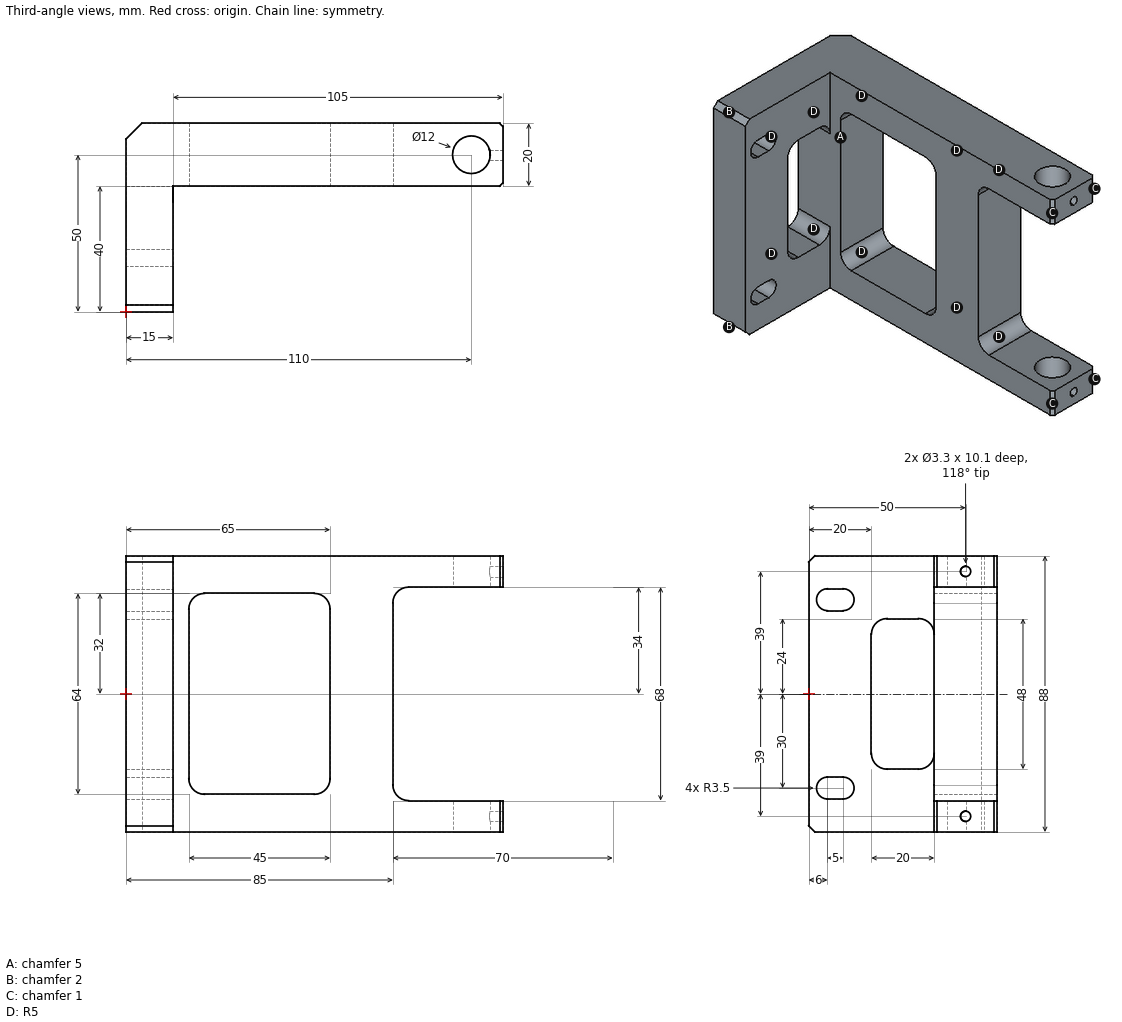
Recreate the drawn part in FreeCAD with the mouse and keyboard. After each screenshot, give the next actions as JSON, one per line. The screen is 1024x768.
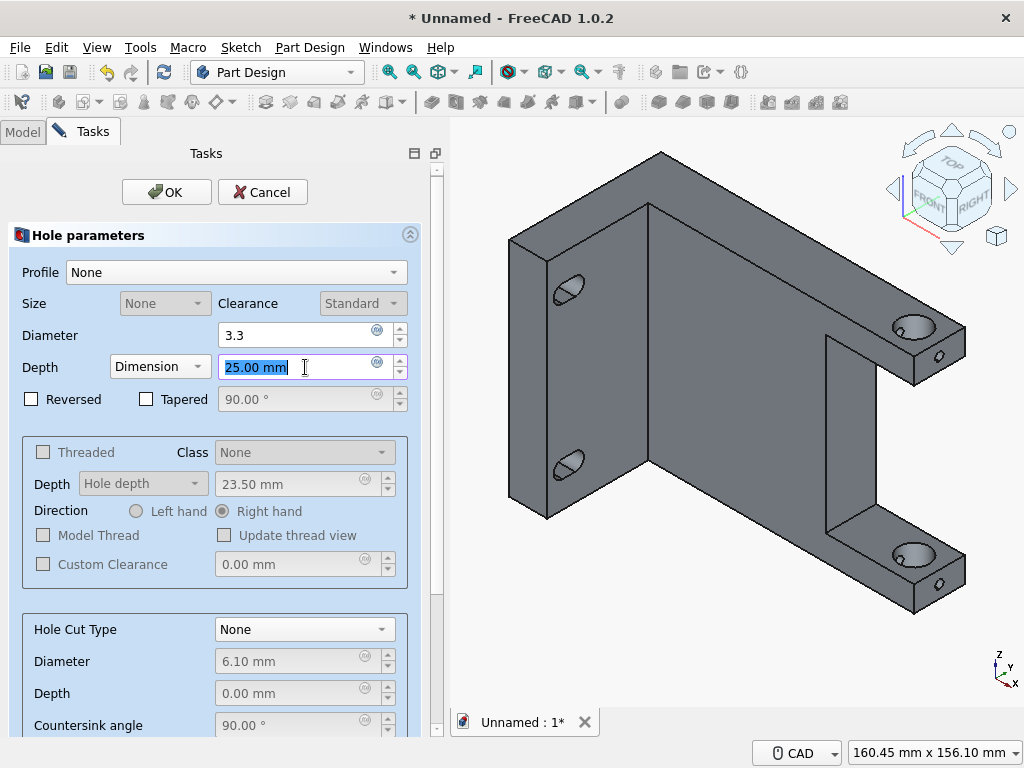
{"action": "type", "text": "10.1"}
{"action": "key", "text": "Tab"}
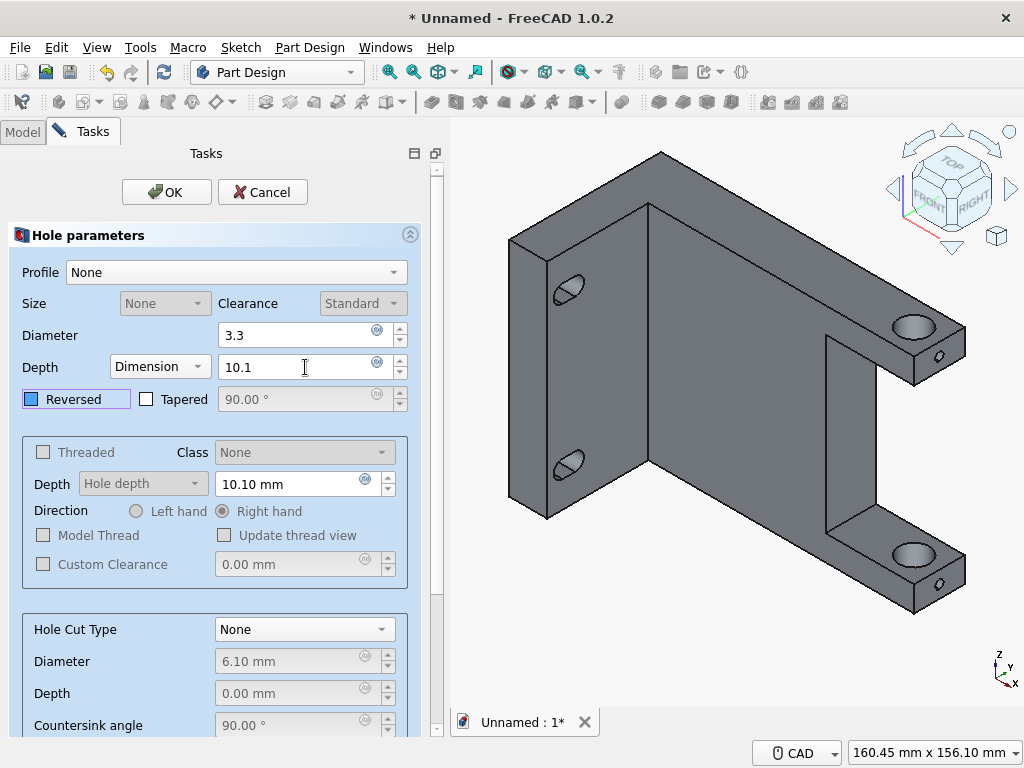
{"action": "left_click", "coordinate": [167, 192]}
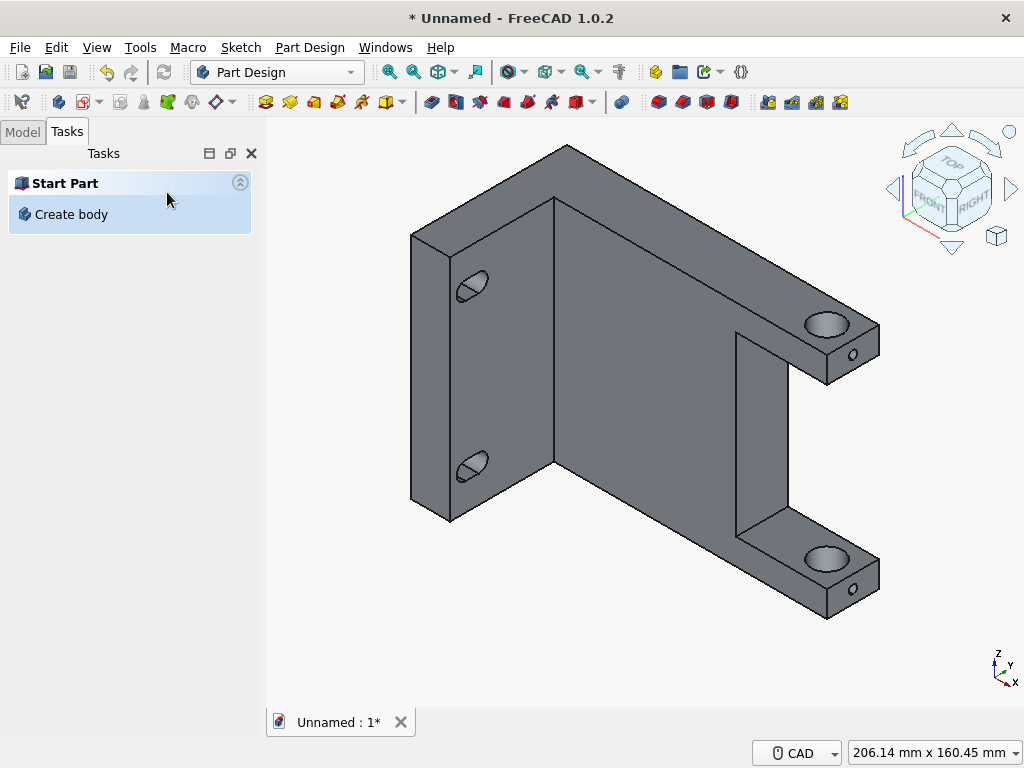
{"action": "key", "text": "4"}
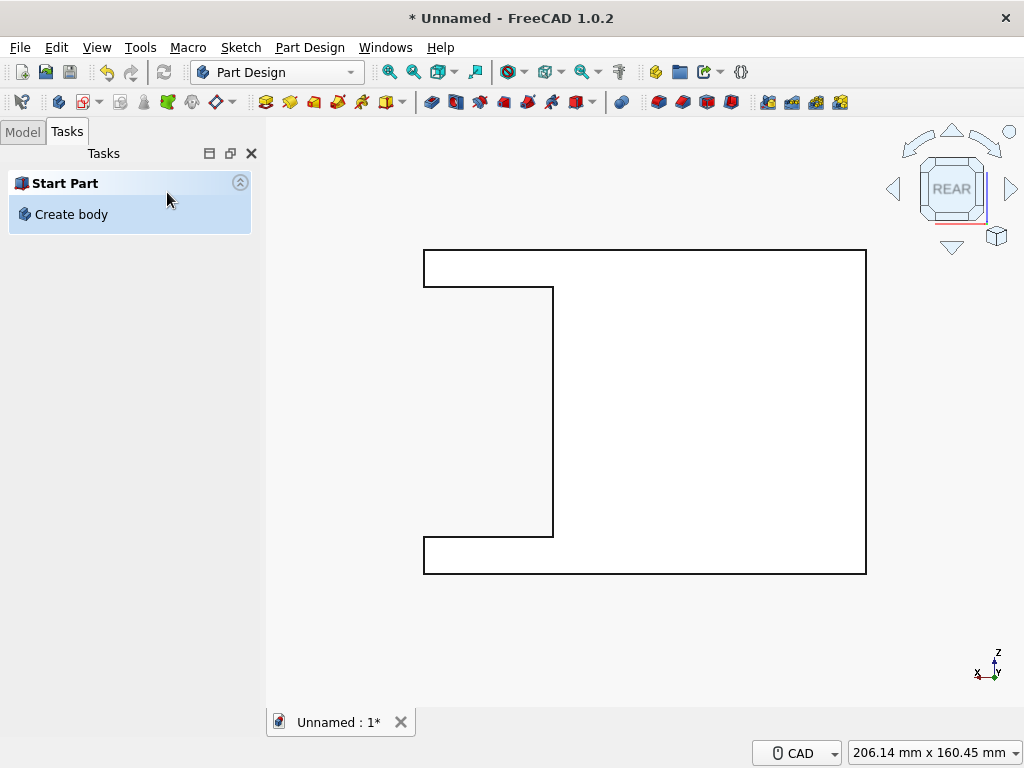
{"action": "left_click", "coordinate": [708, 411]}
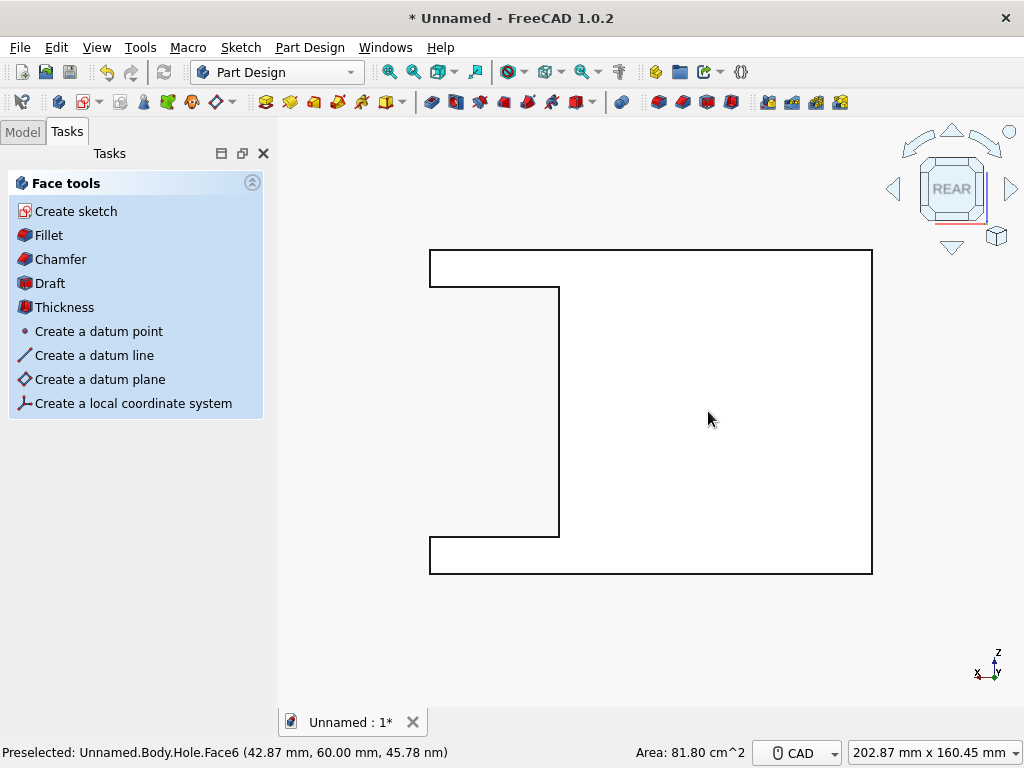
{"action": "left_click", "coordinate": [84, 102]}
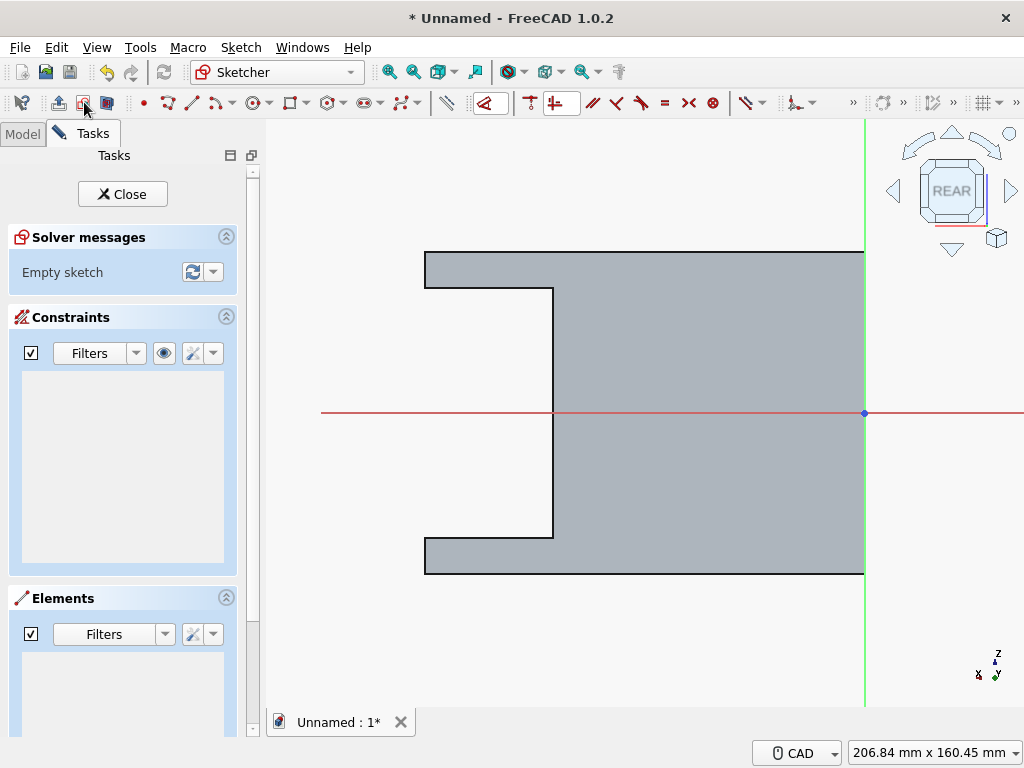
{"action": "scroll", "coordinate": [294, 413], "scroll_direction": "down", "scroll_amount": 1}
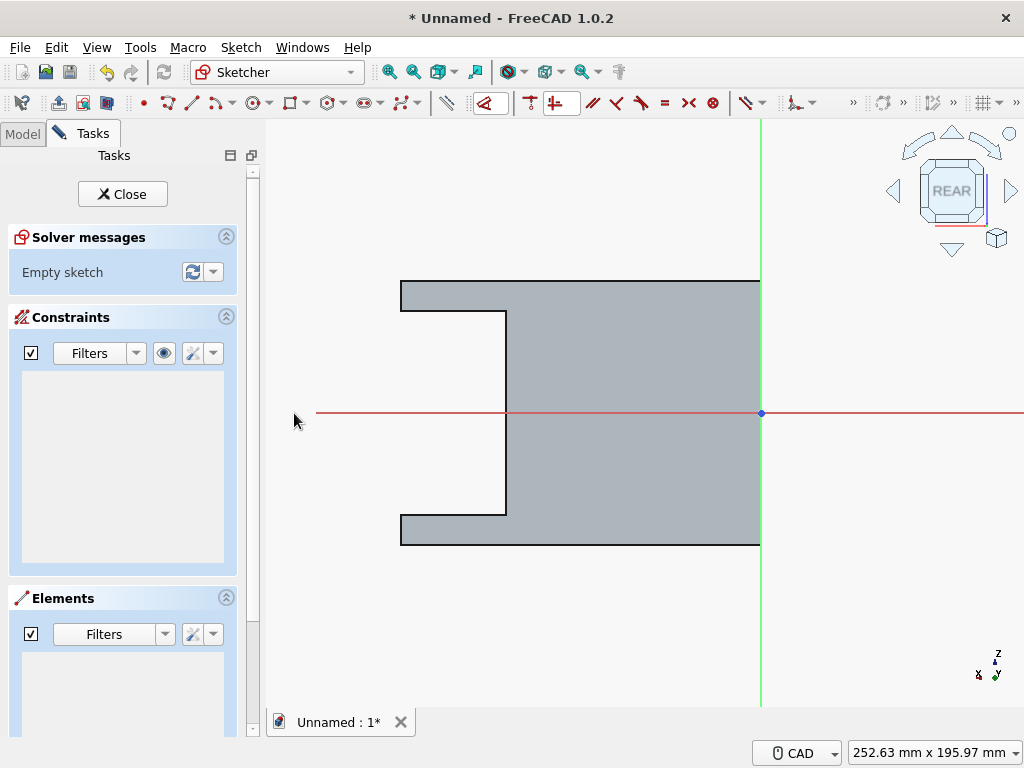
{"action": "scroll", "coordinate": [770, 413], "scroll_direction": "up", "scroll_amount": 3}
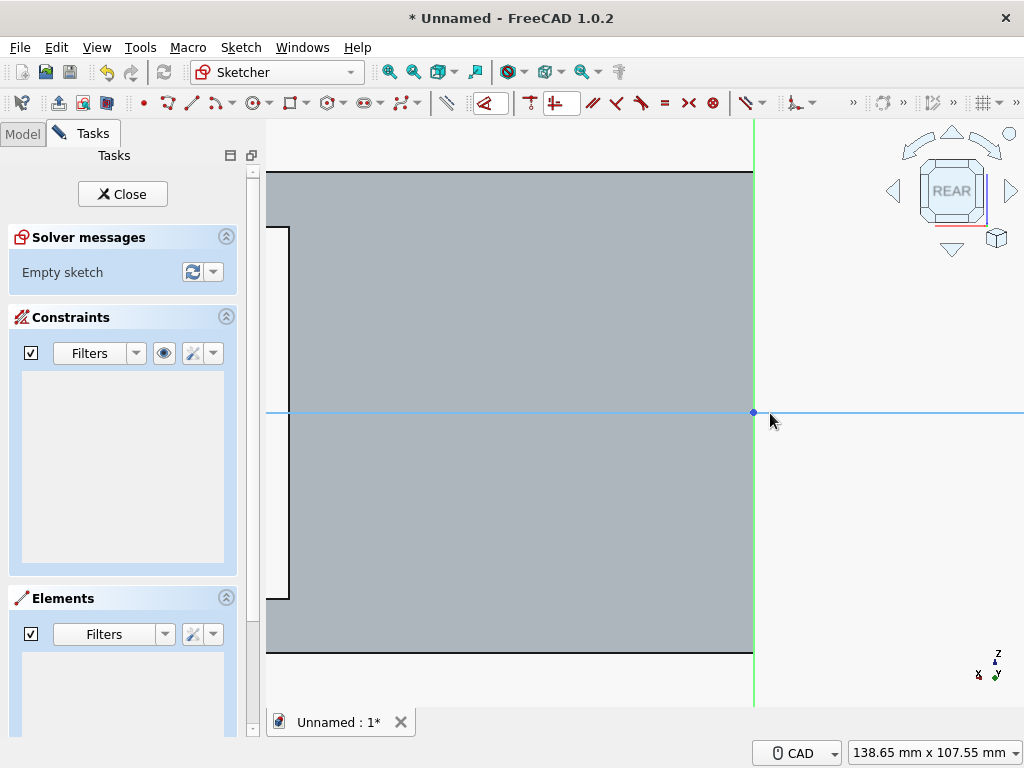
{"action": "left_click", "coordinate": [290, 104]}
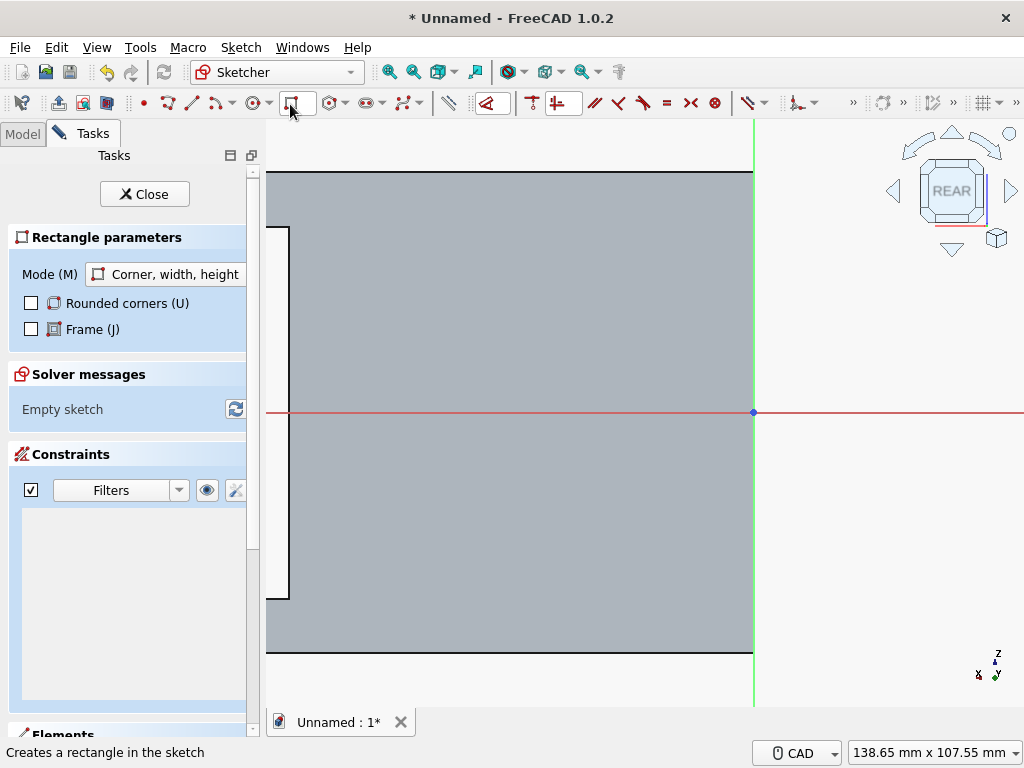
{"action": "left_click", "coordinate": [398, 238]}
{"action": "mouse_move", "coordinate": [644, 588]}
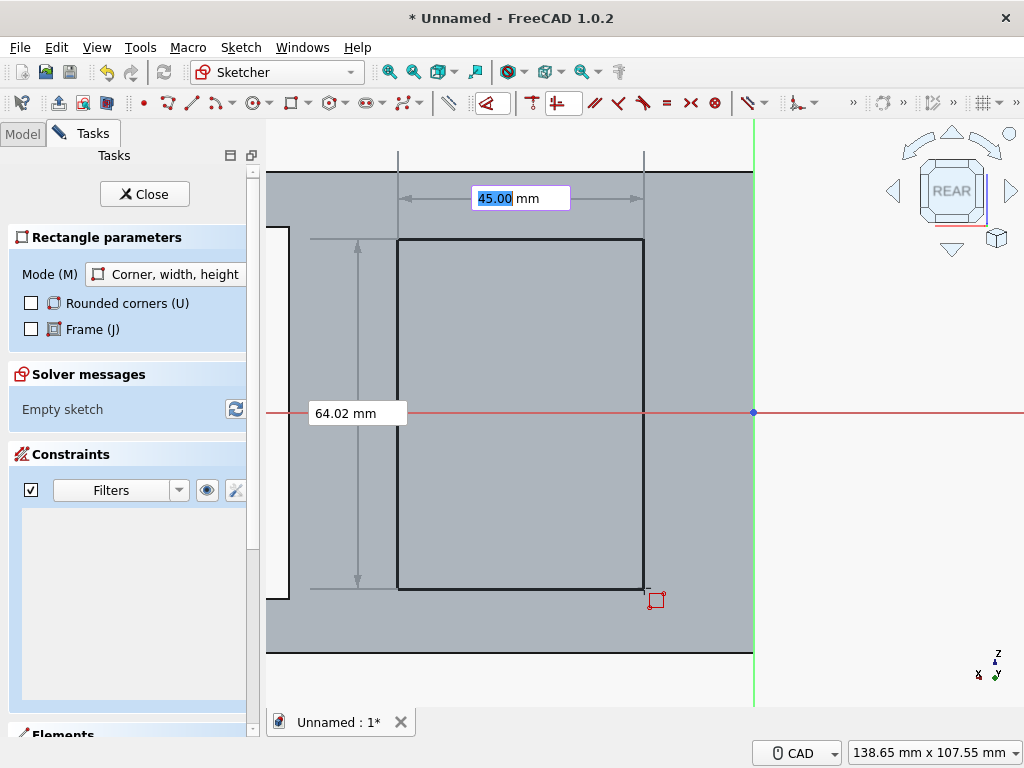
{"action": "type", "text": "45"}
{"action": "key", "text": "Tab"}
{"action": "type", "text": "64"}
{"action": "key", "text": "Return"}
{"action": "key", "text": "Escape"}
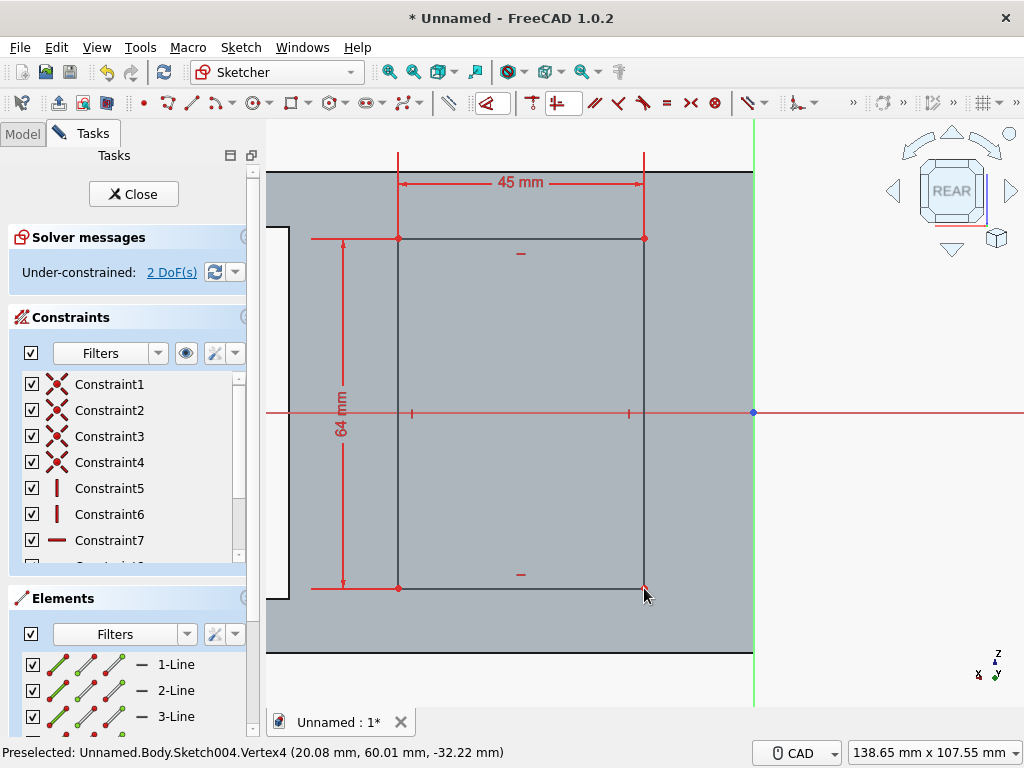
{"action": "left_click", "coordinate": [398, 239]}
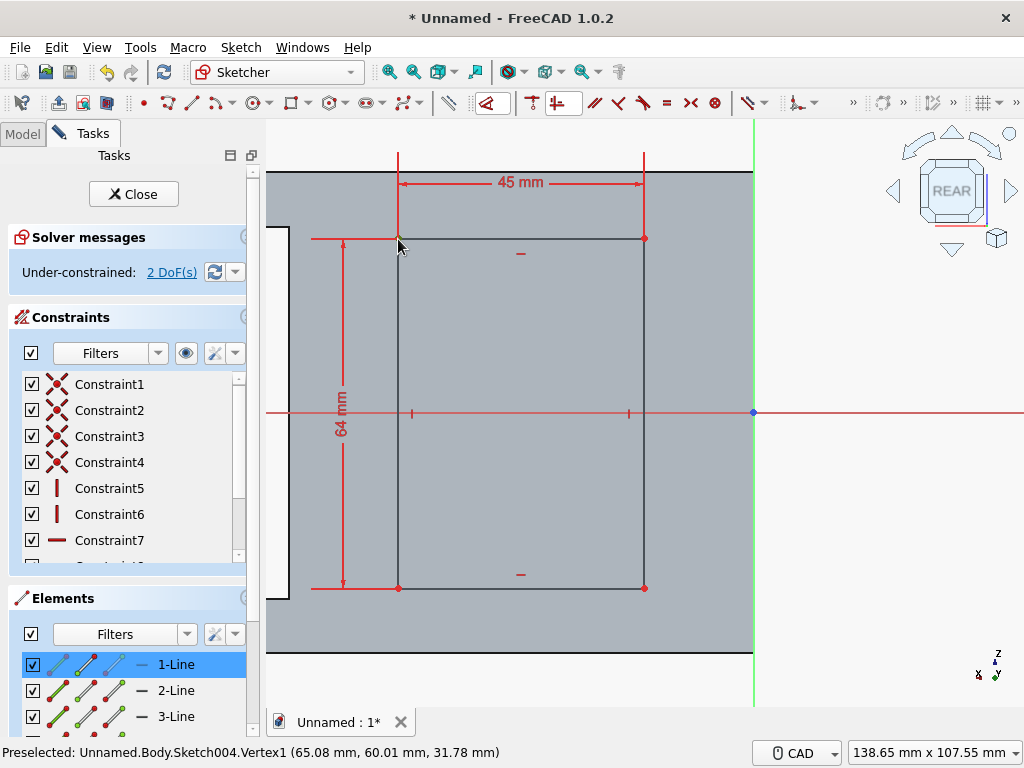
{"action": "left_click", "coordinate": [504, 104]}